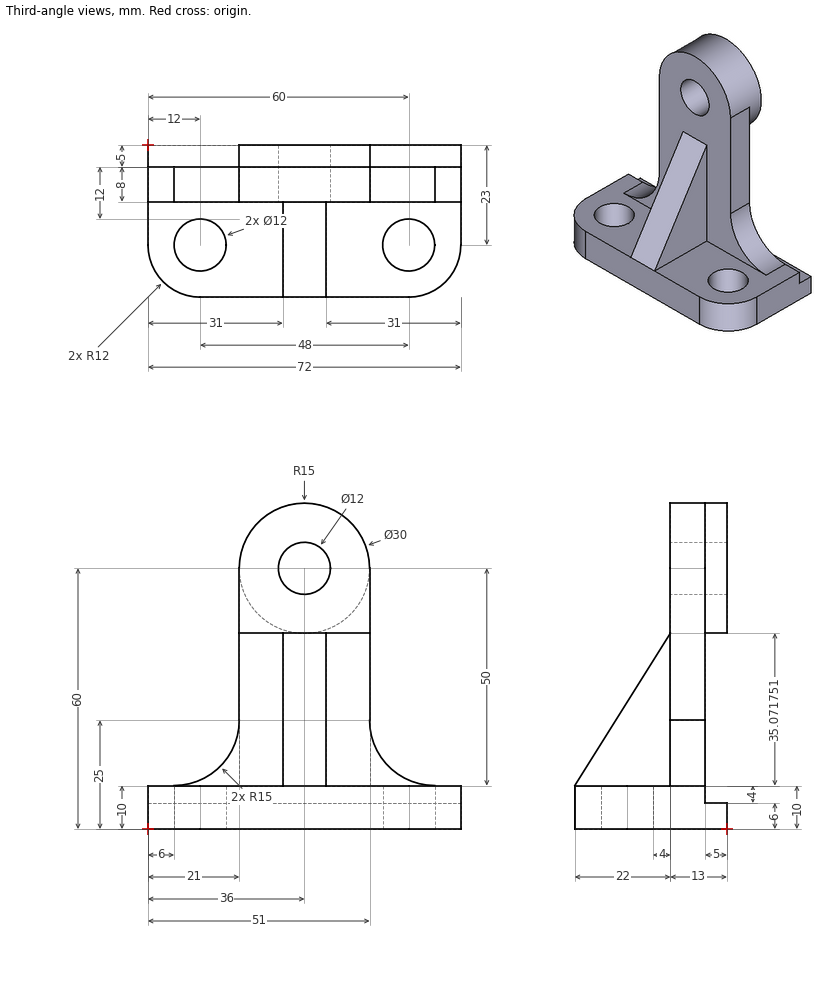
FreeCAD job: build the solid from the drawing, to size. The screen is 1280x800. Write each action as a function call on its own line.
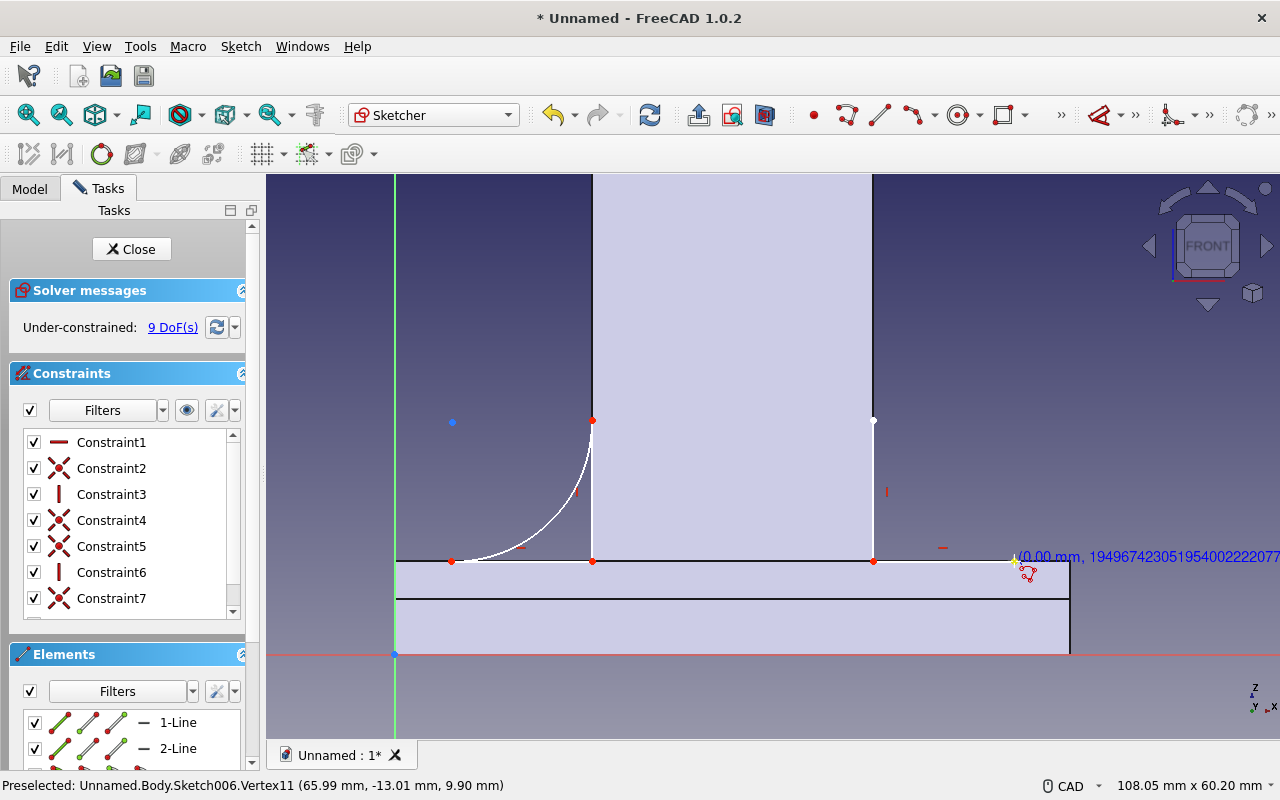
key(g)
key(3)
key(a)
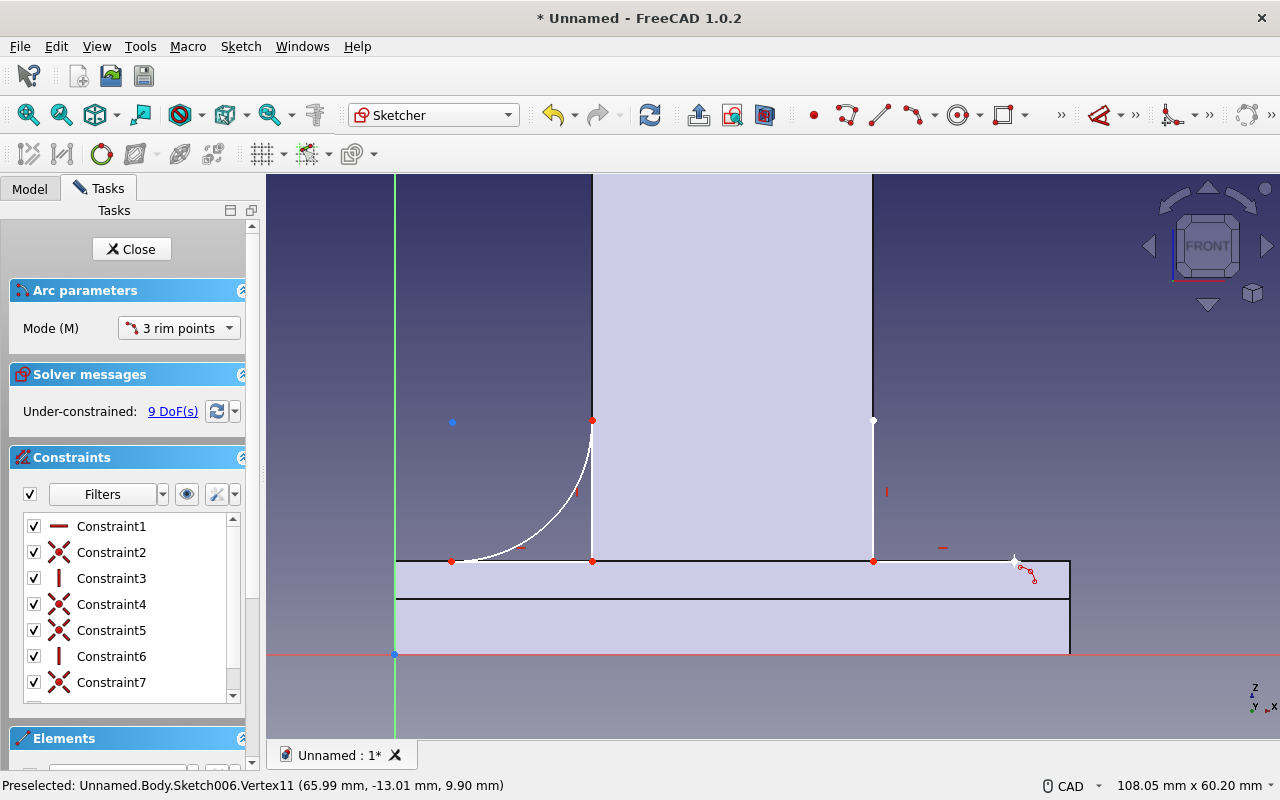
click(1014, 562)
click(873, 421)
click(915, 520)
key(Escape)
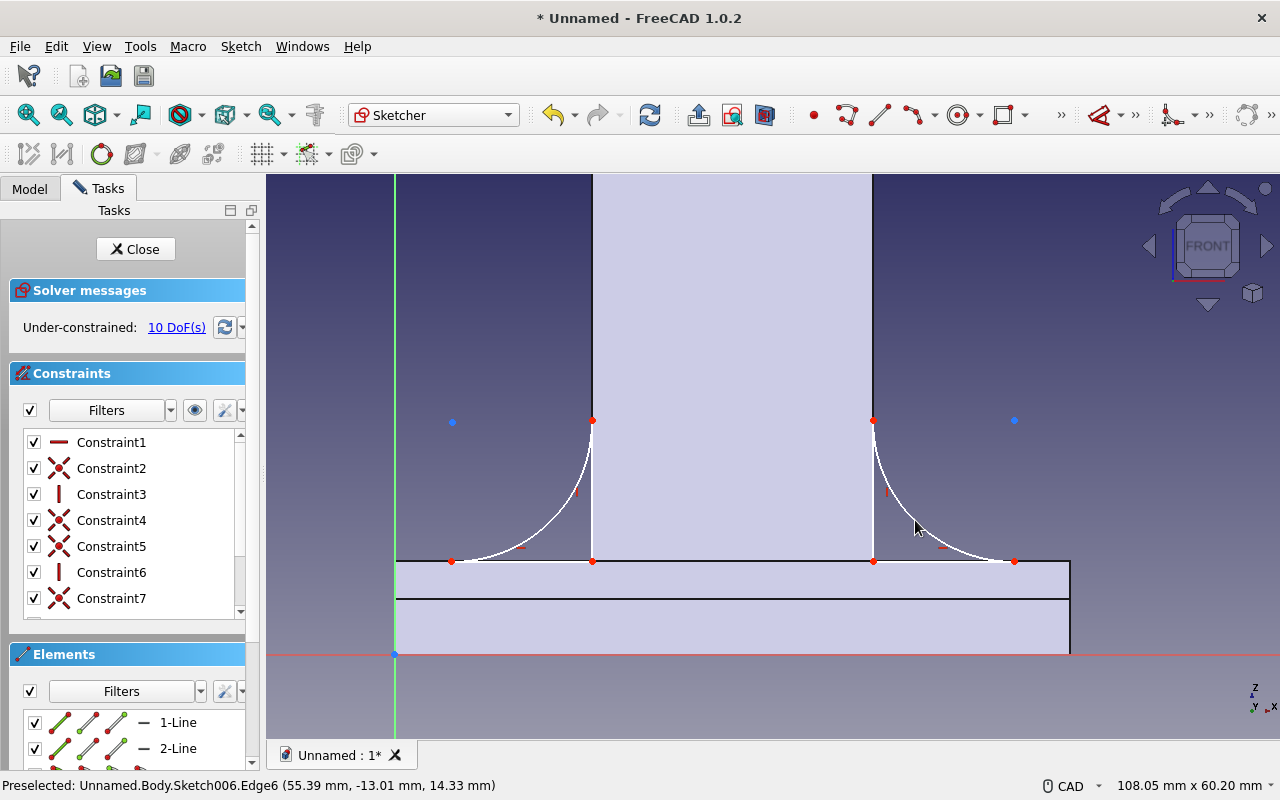
click(550, 562)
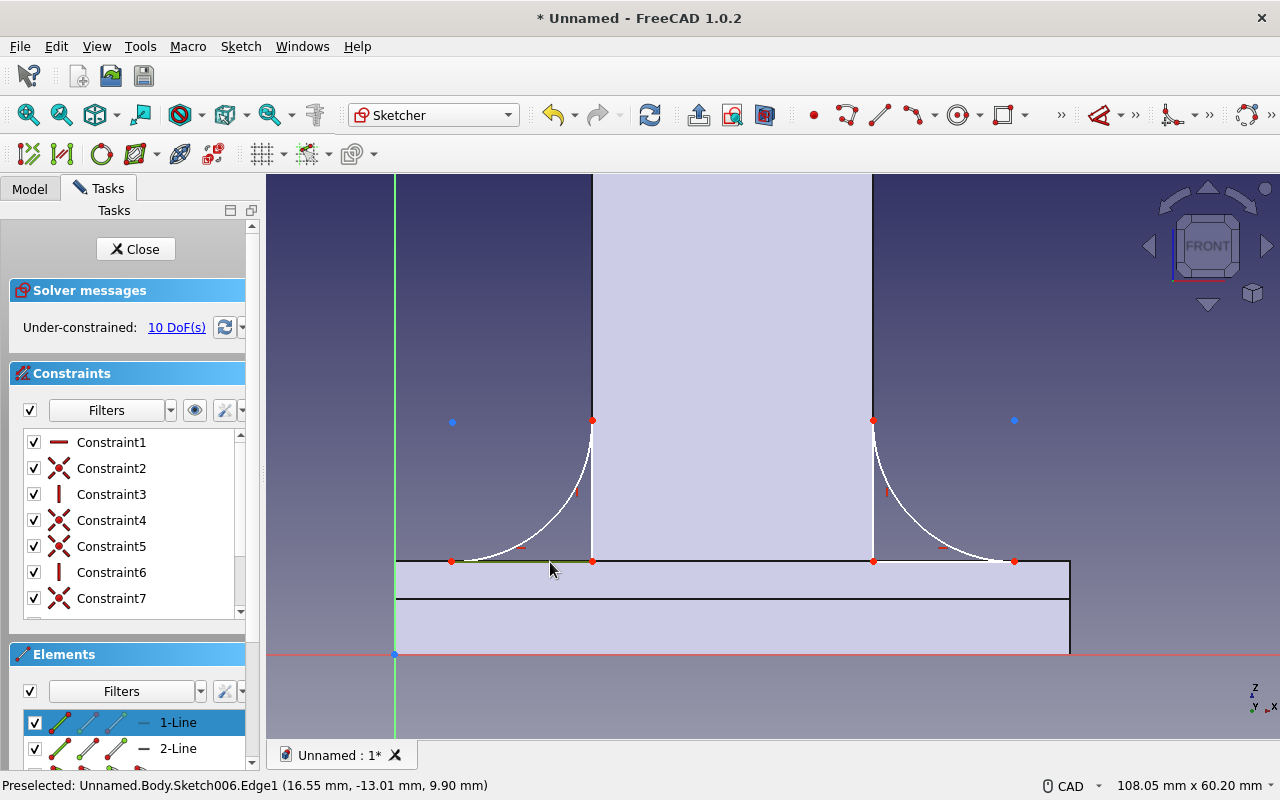
click(515, 547)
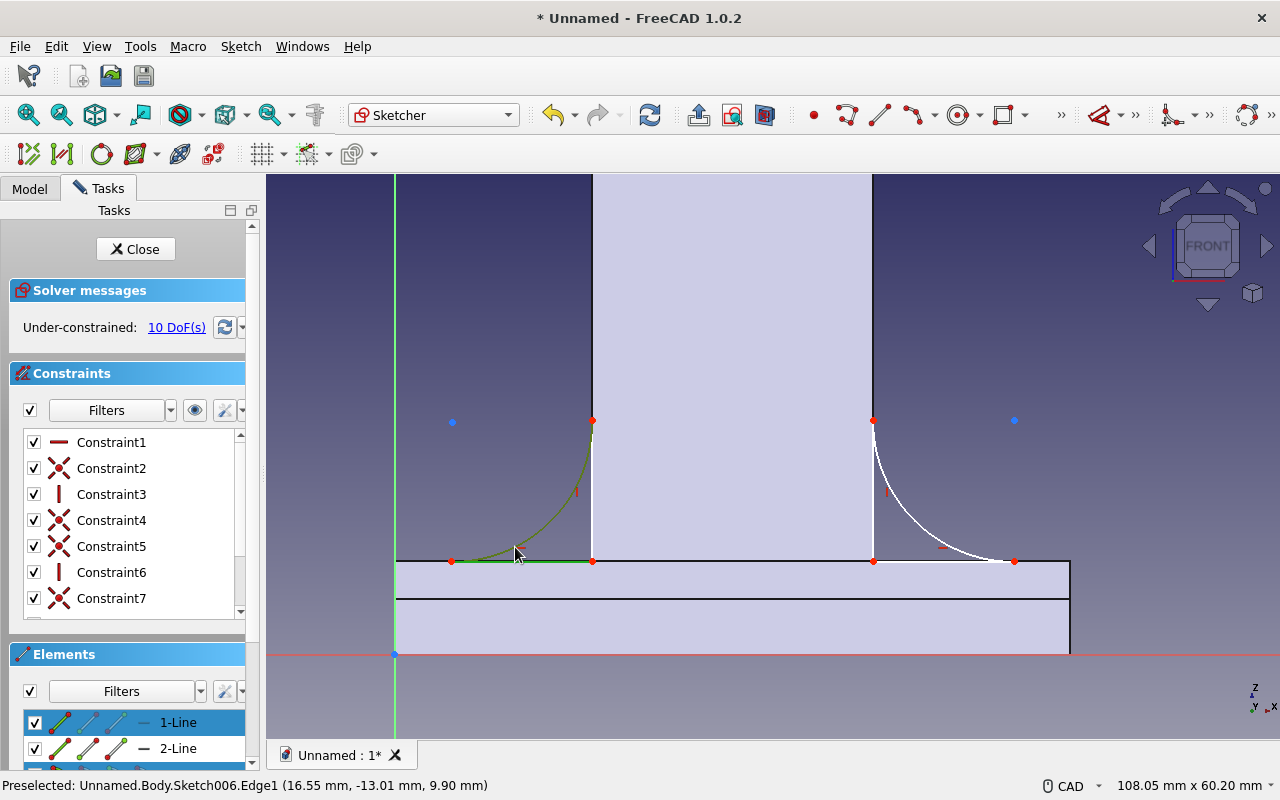
key(t)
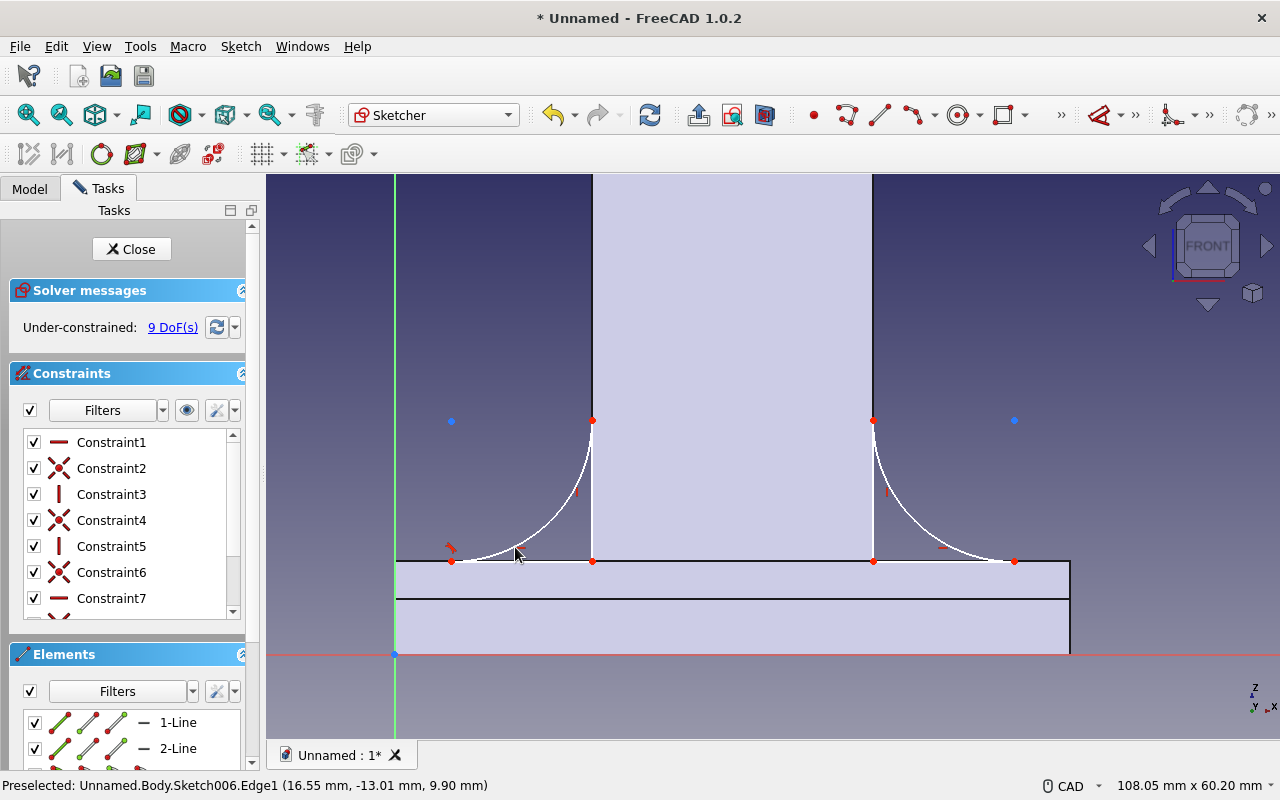
click(592, 520)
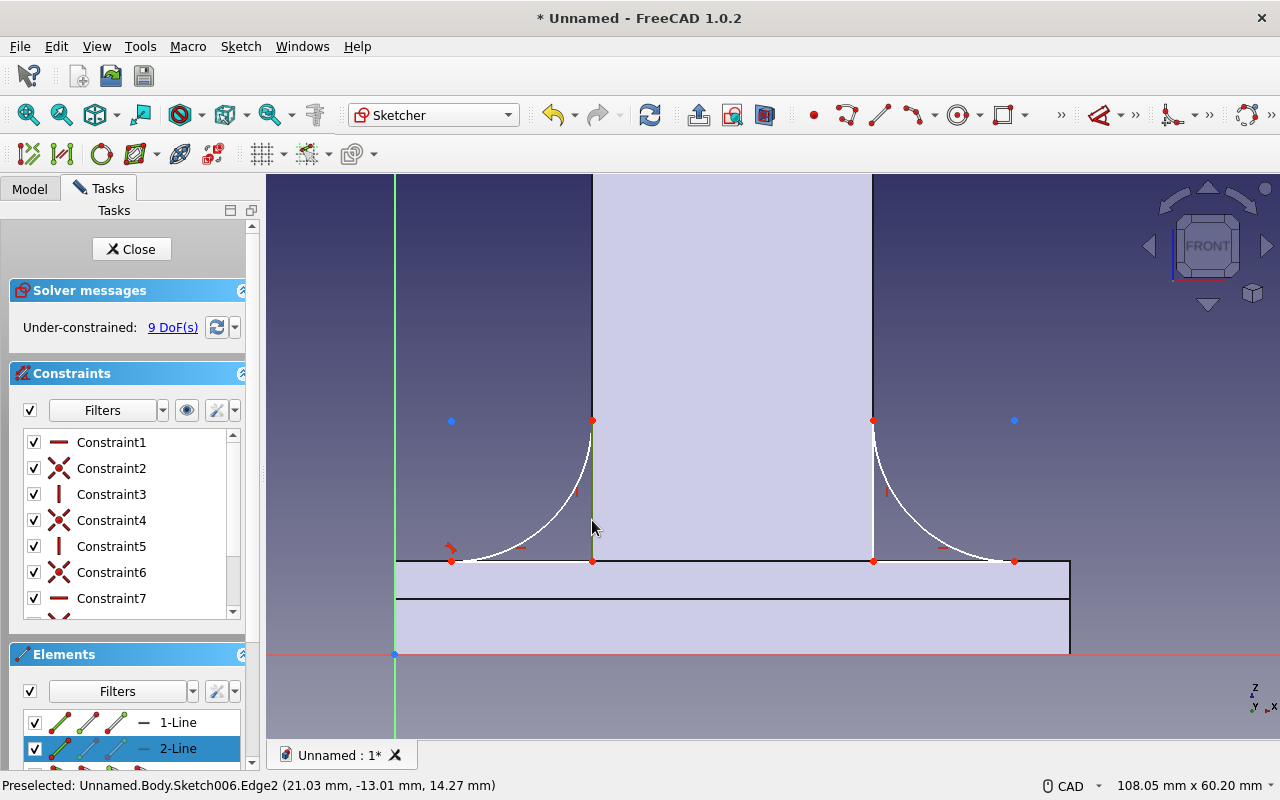
click(515, 547)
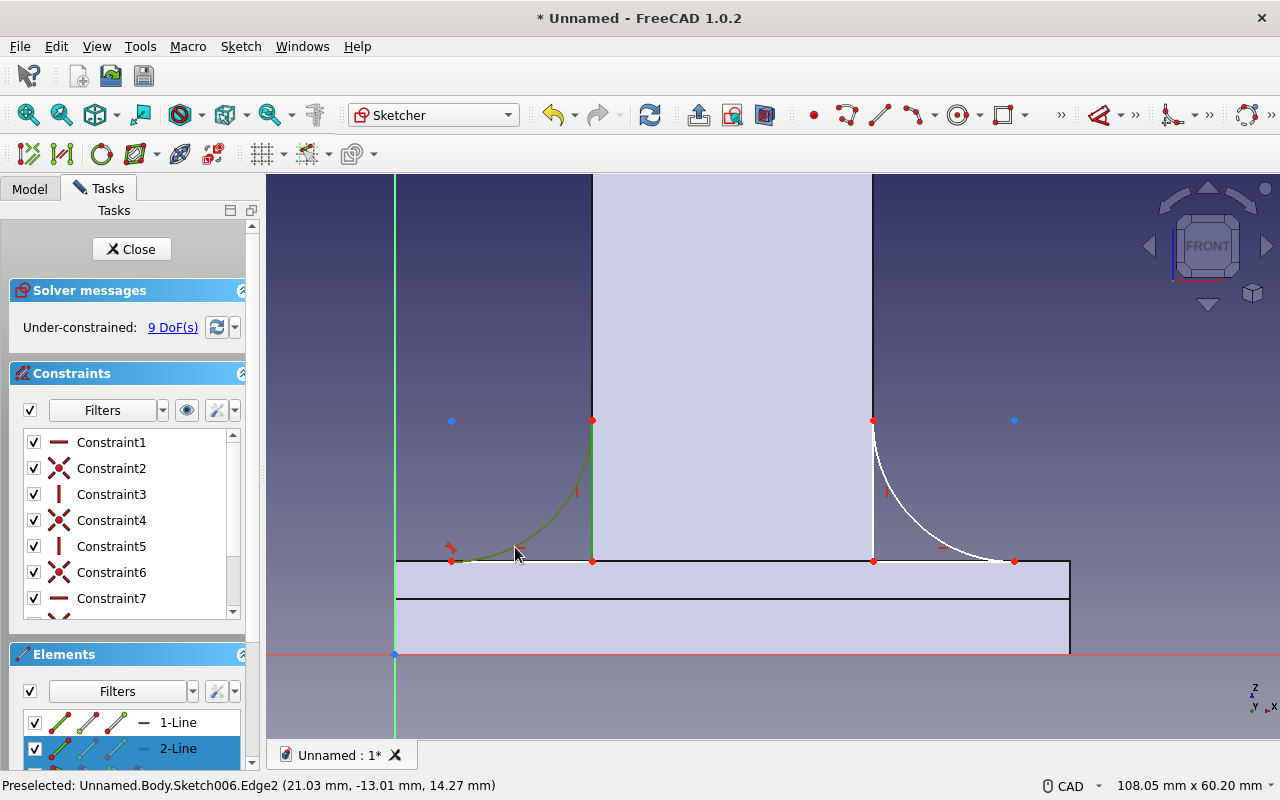
key(t)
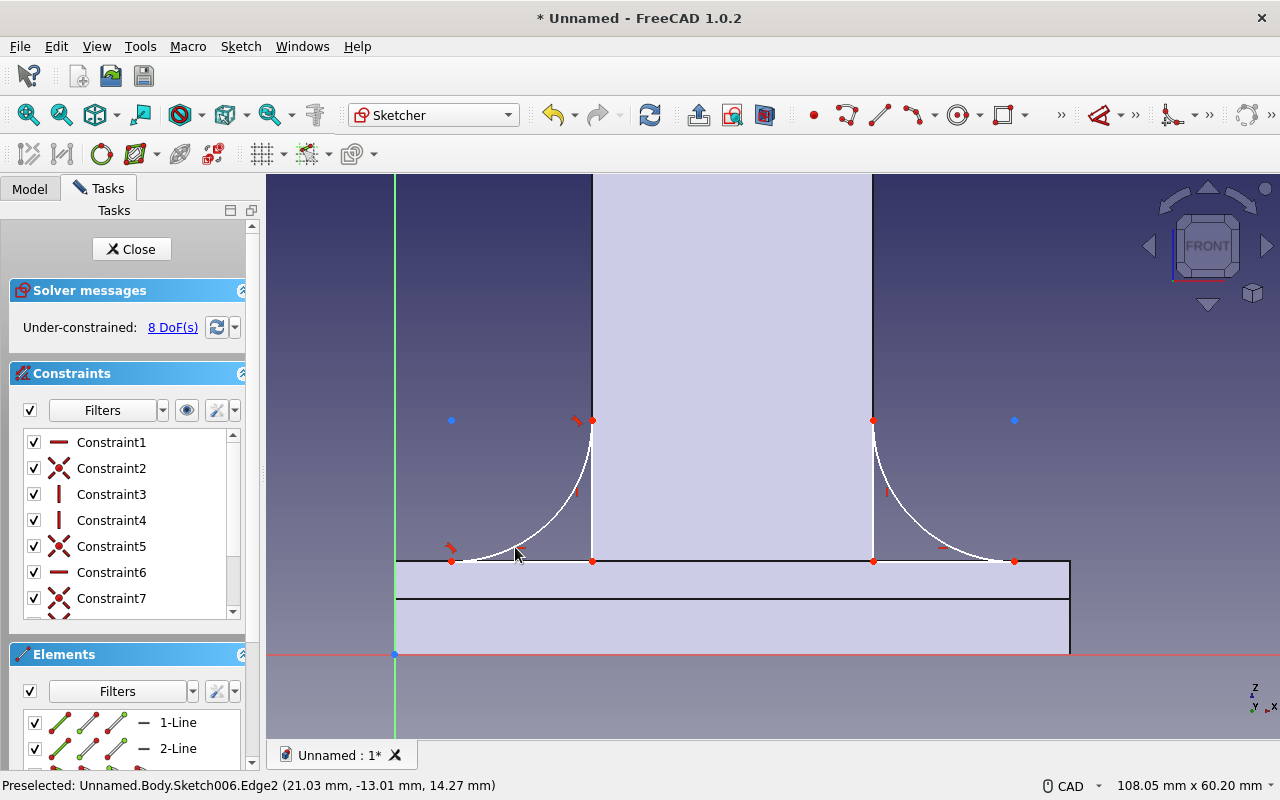
click(873, 520)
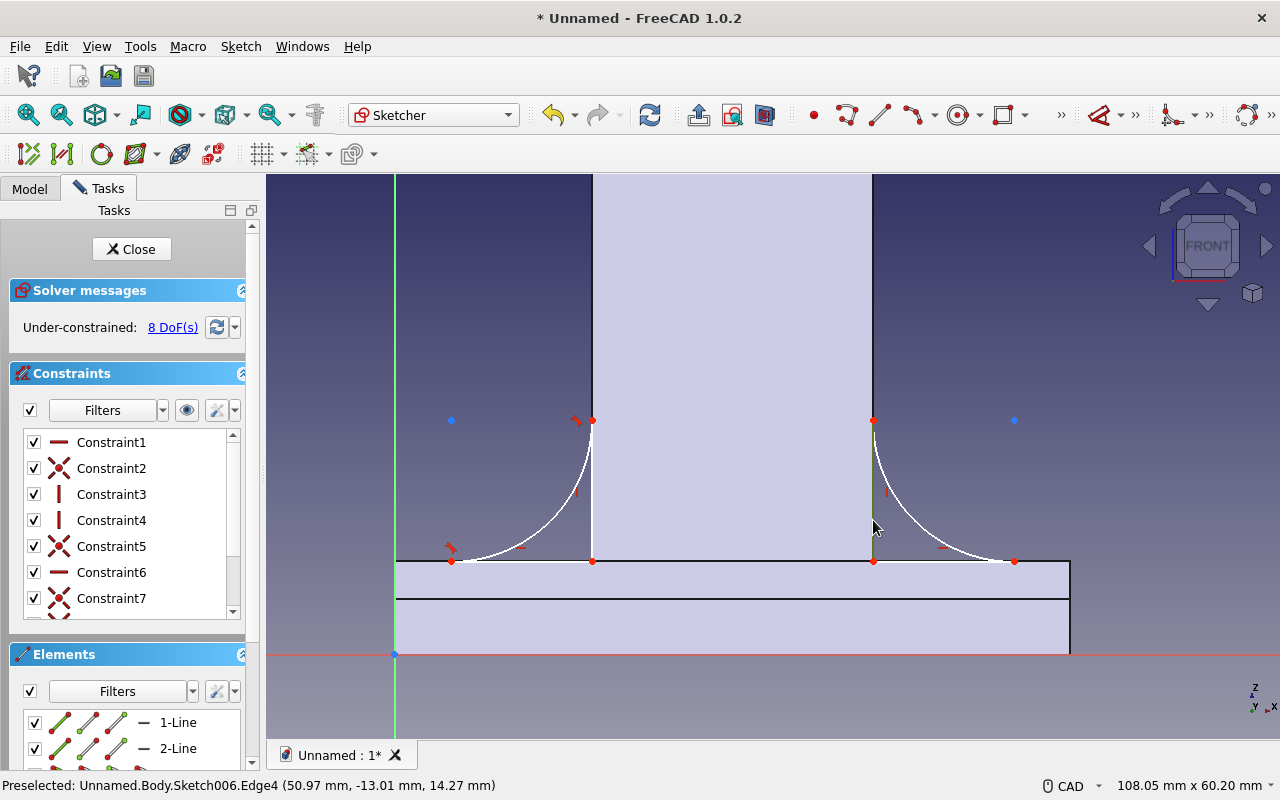
click(950, 546)